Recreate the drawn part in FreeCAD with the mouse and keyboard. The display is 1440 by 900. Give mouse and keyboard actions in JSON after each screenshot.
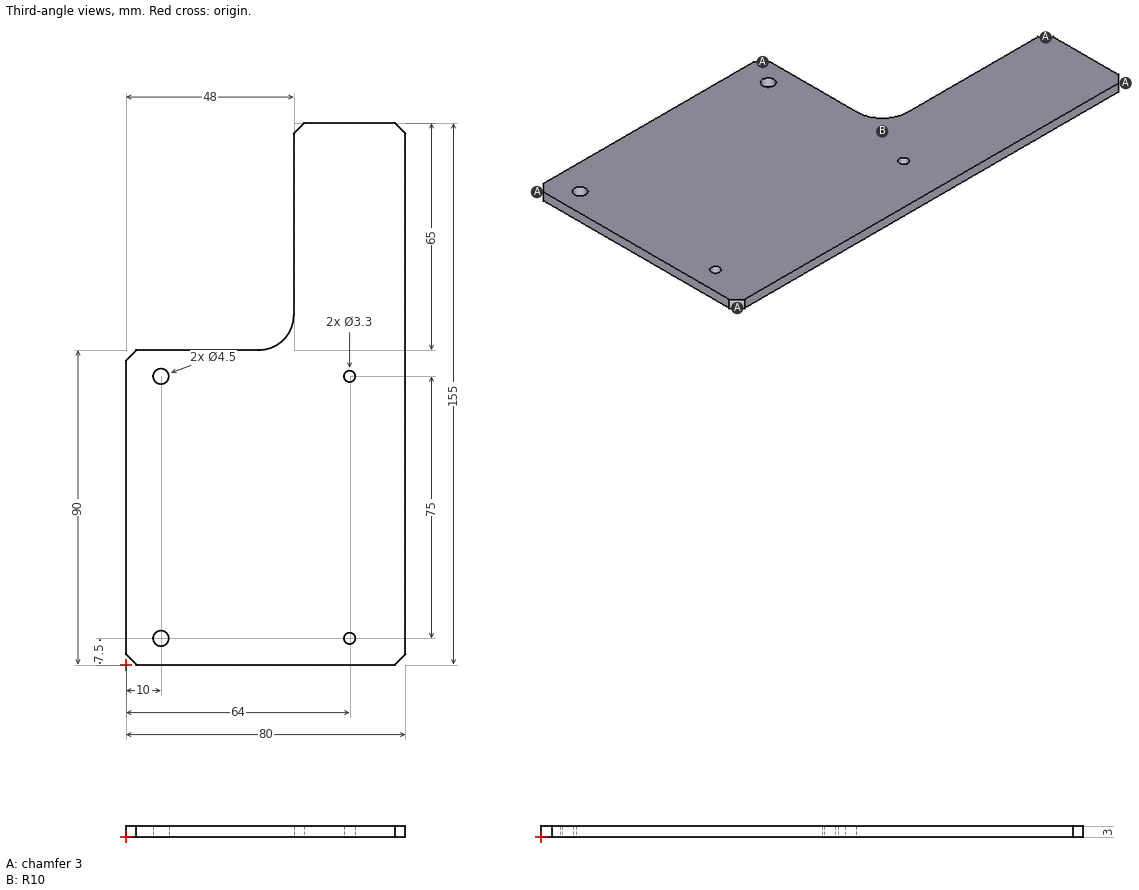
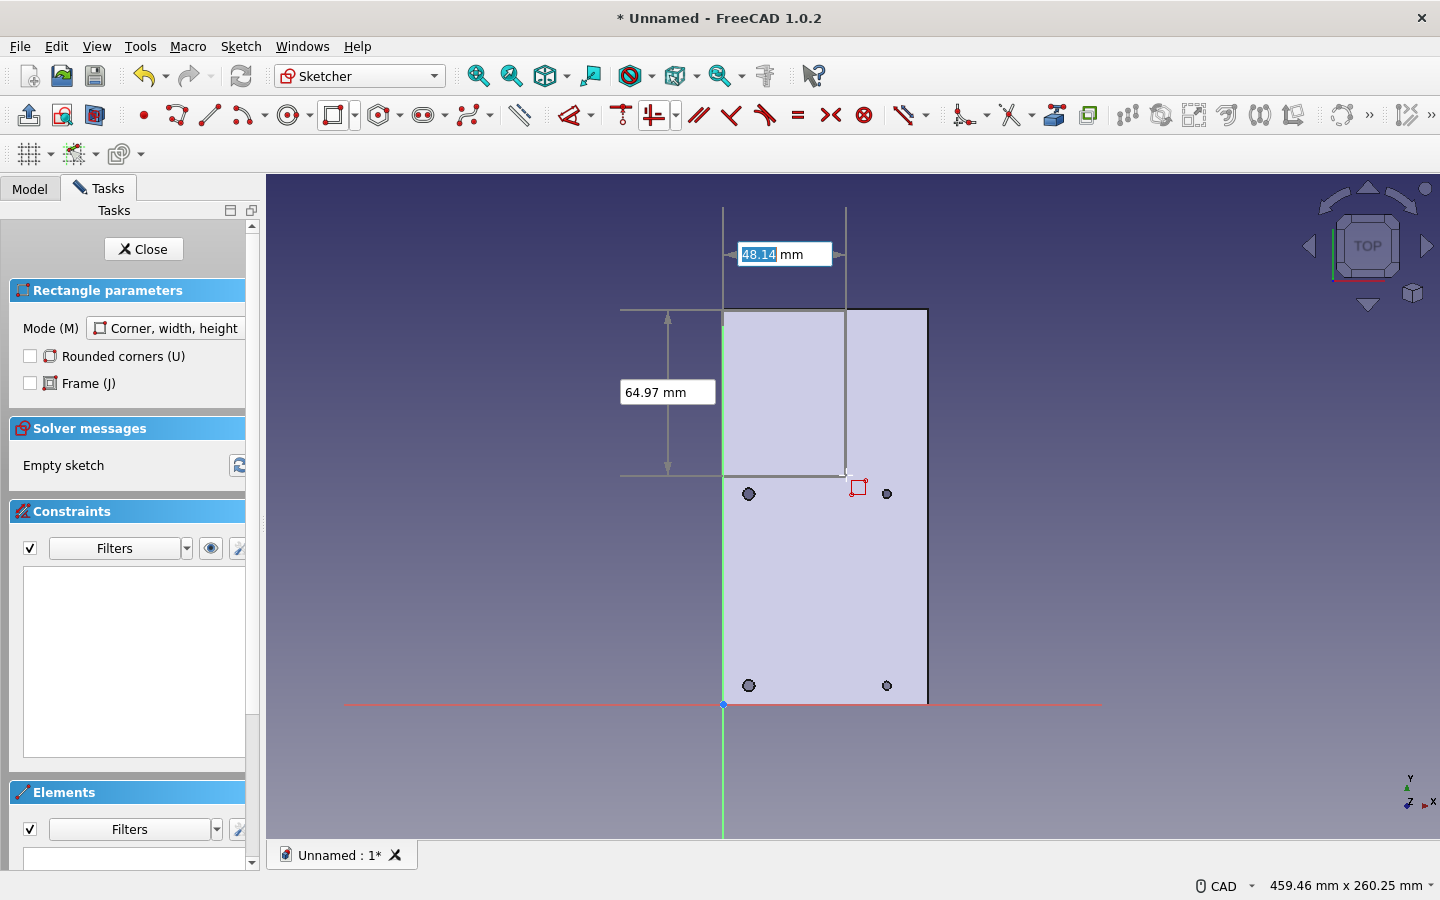
{"action": "type", "text": "48"}
{"action": "key", "text": "Tab"}
{"action": "type", "text": "65"}
{"action": "key", "text": "Return"}
{"action": "key", "text": "Escape"}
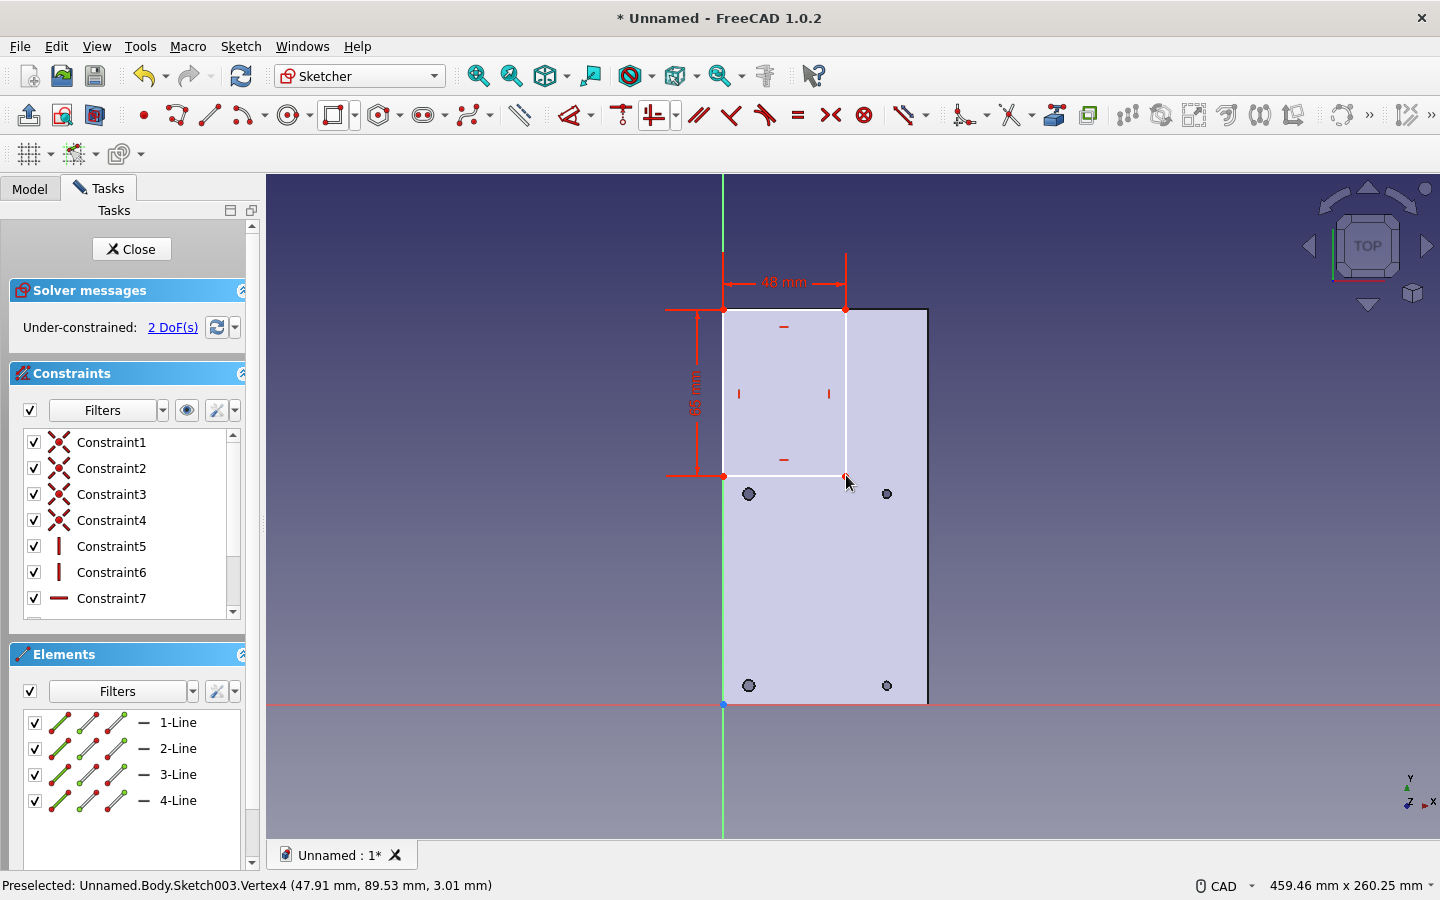
{"action": "left_click", "coordinate": [723, 310]}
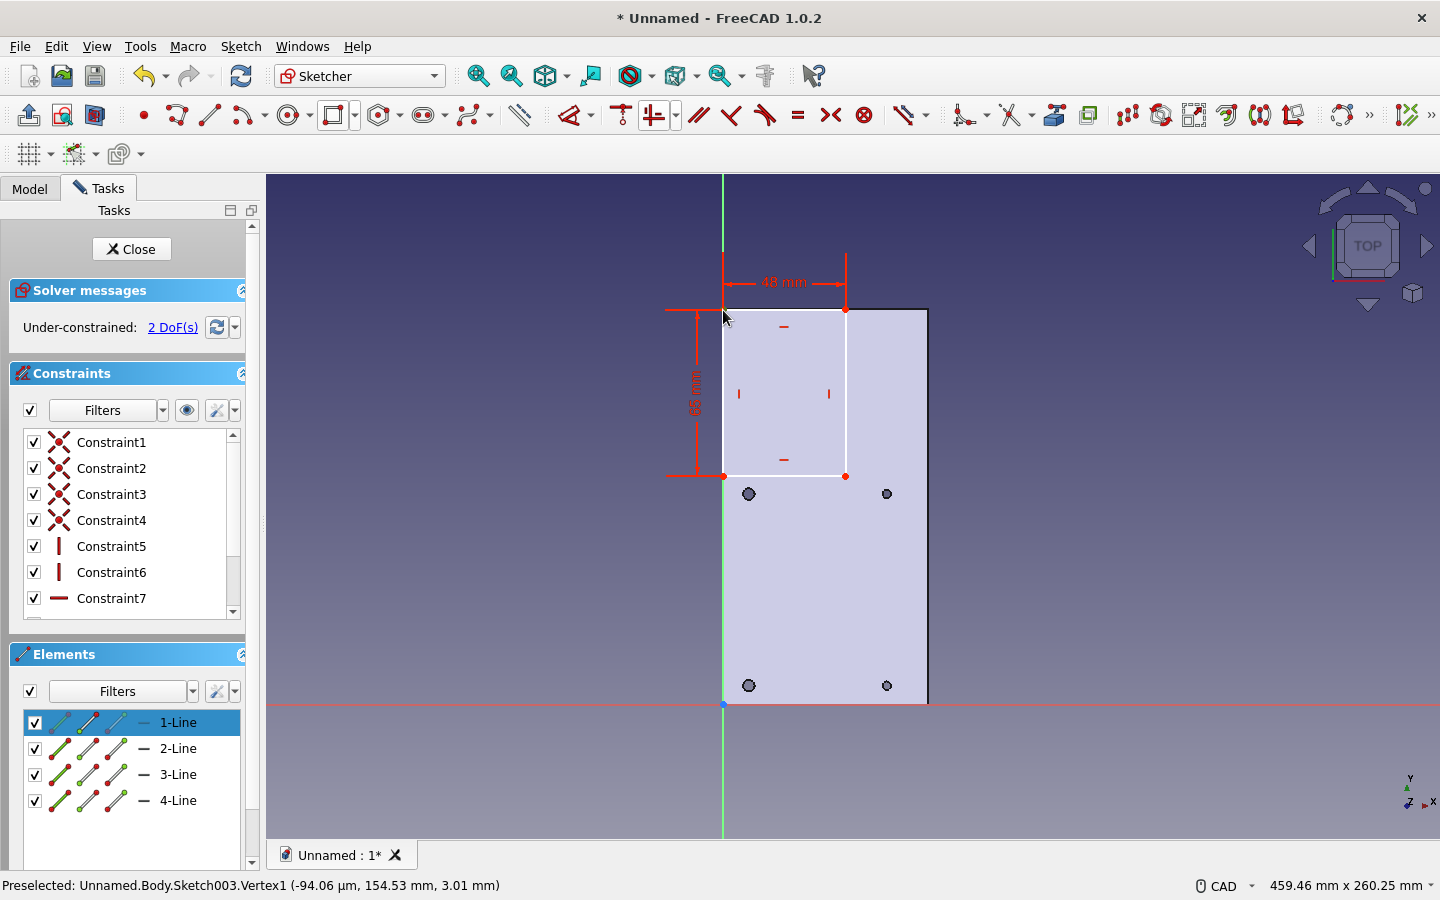
{"action": "left_click", "coordinate": [723, 768]}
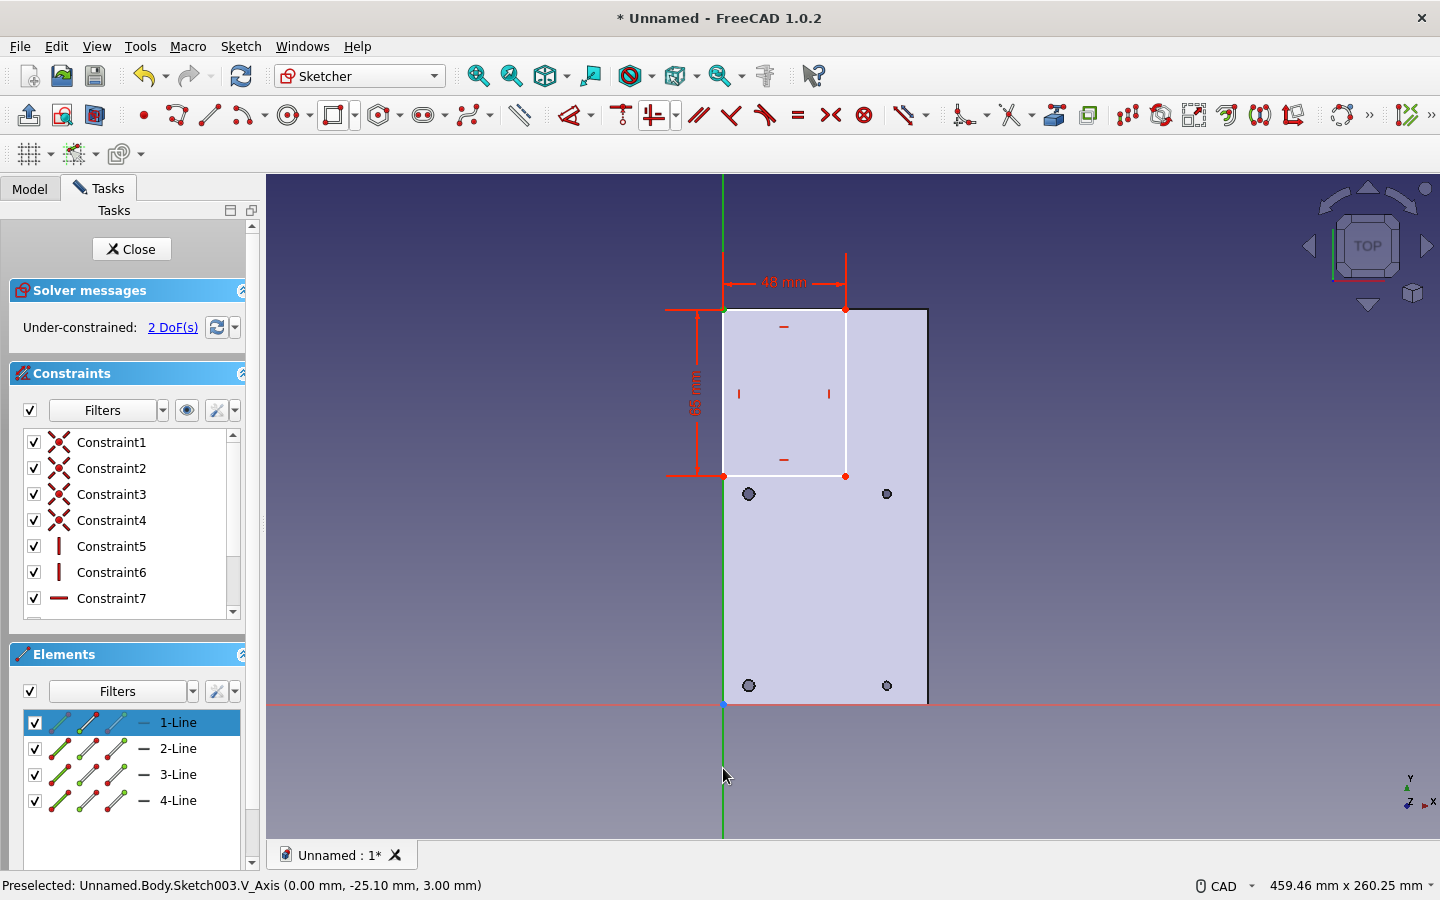
{"action": "key", "text": "c"}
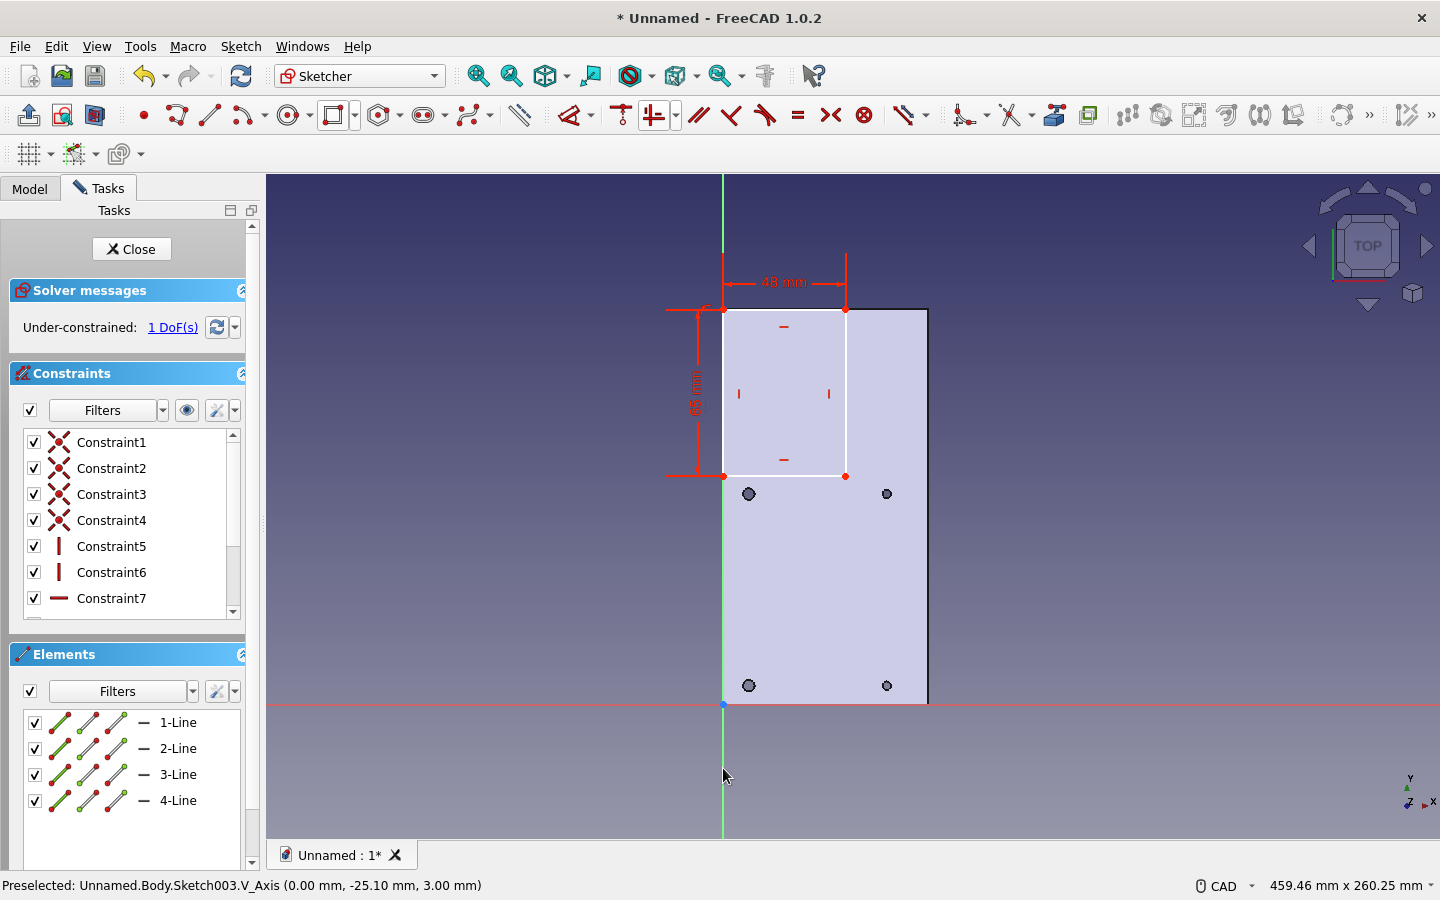
{"action": "left_click", "coordinate": [568, 116]}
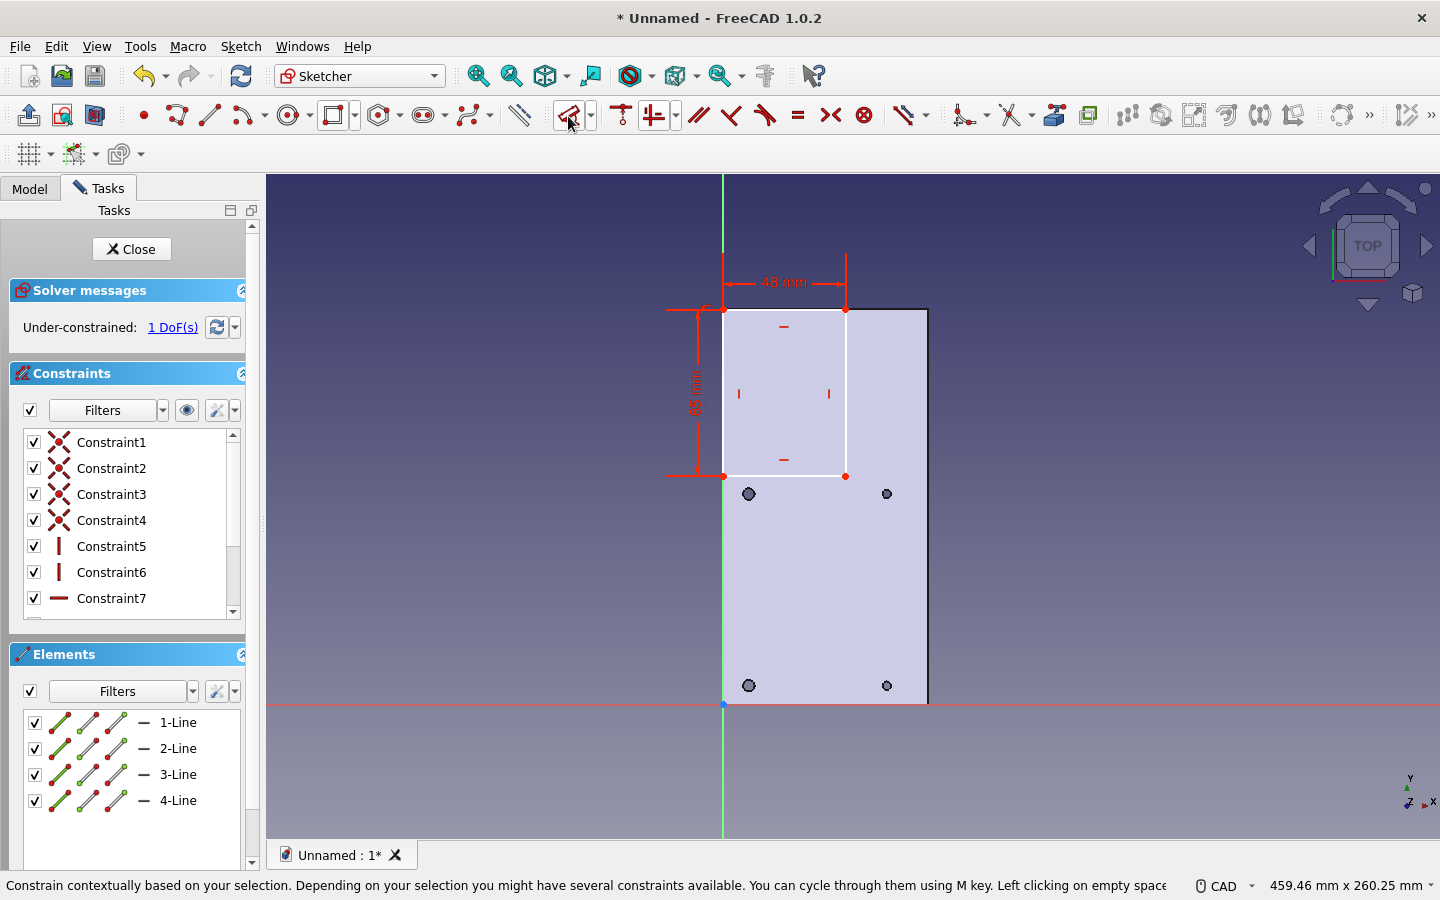
{"action": "left_click", "coordinate": [723, 476]}
{"action": "left_click", "coordinate": [689, 590]}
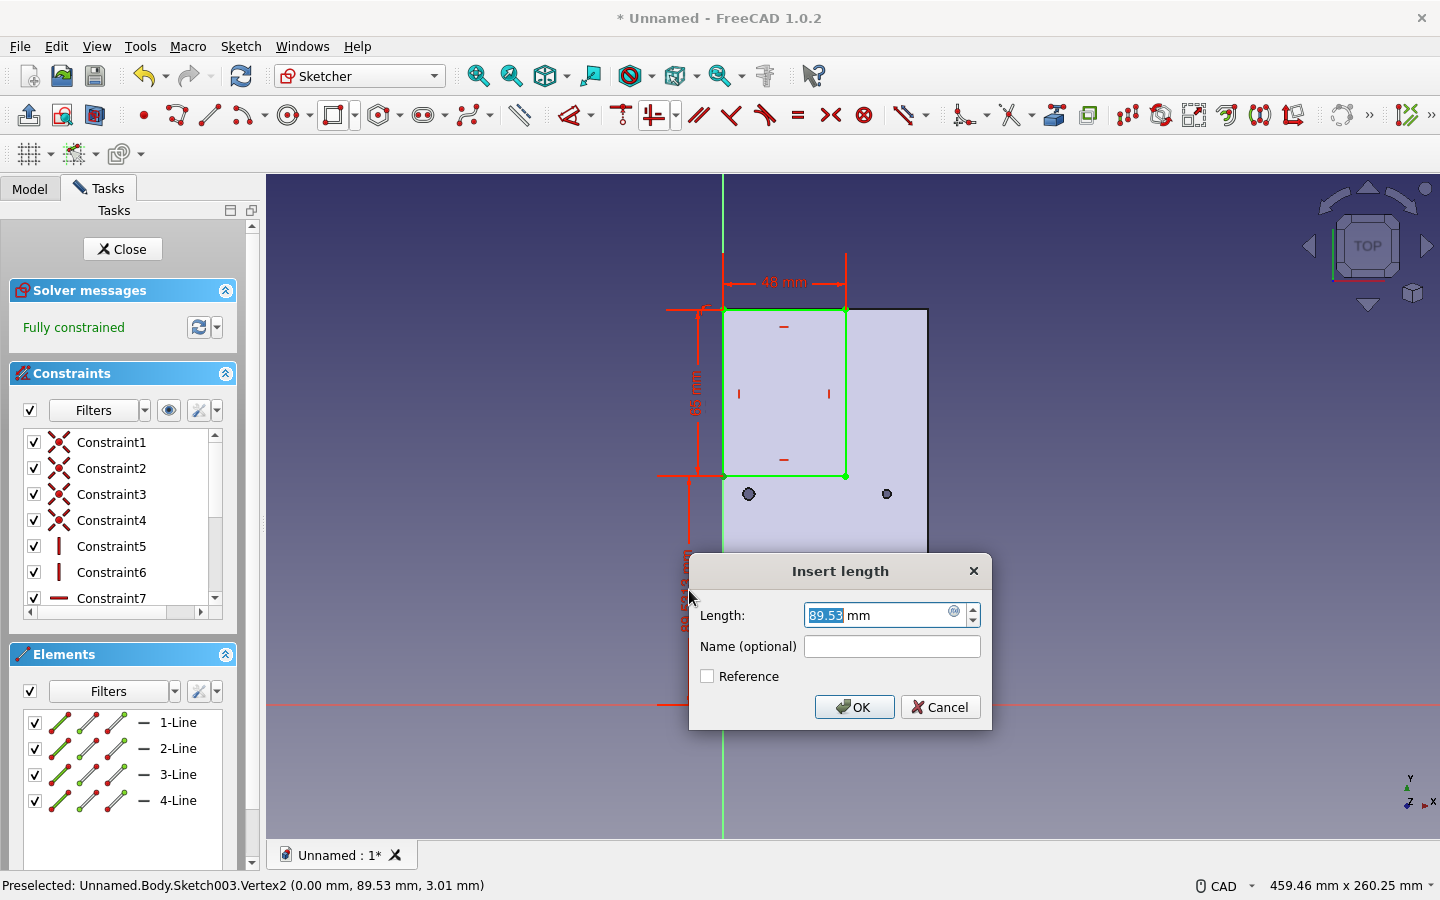
{"action": "type", "text": "90"}
{"action": "key", "text": "Return"}
{"action": "key", "text": "Escape"}